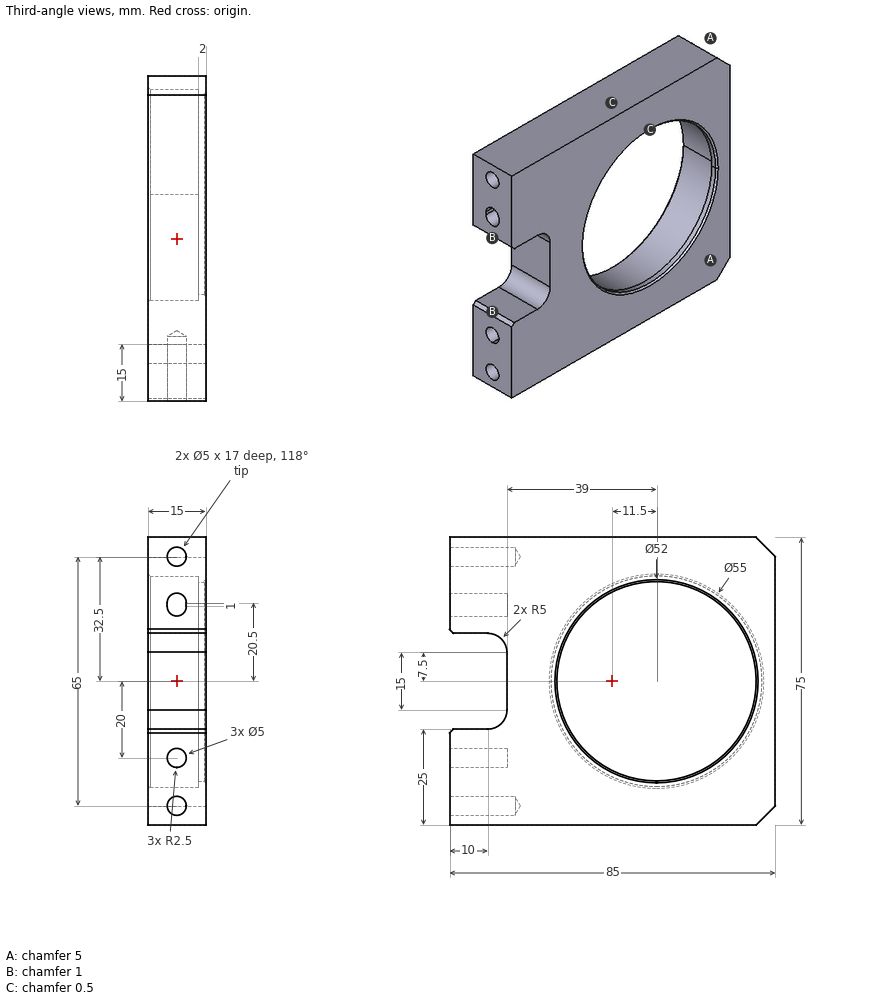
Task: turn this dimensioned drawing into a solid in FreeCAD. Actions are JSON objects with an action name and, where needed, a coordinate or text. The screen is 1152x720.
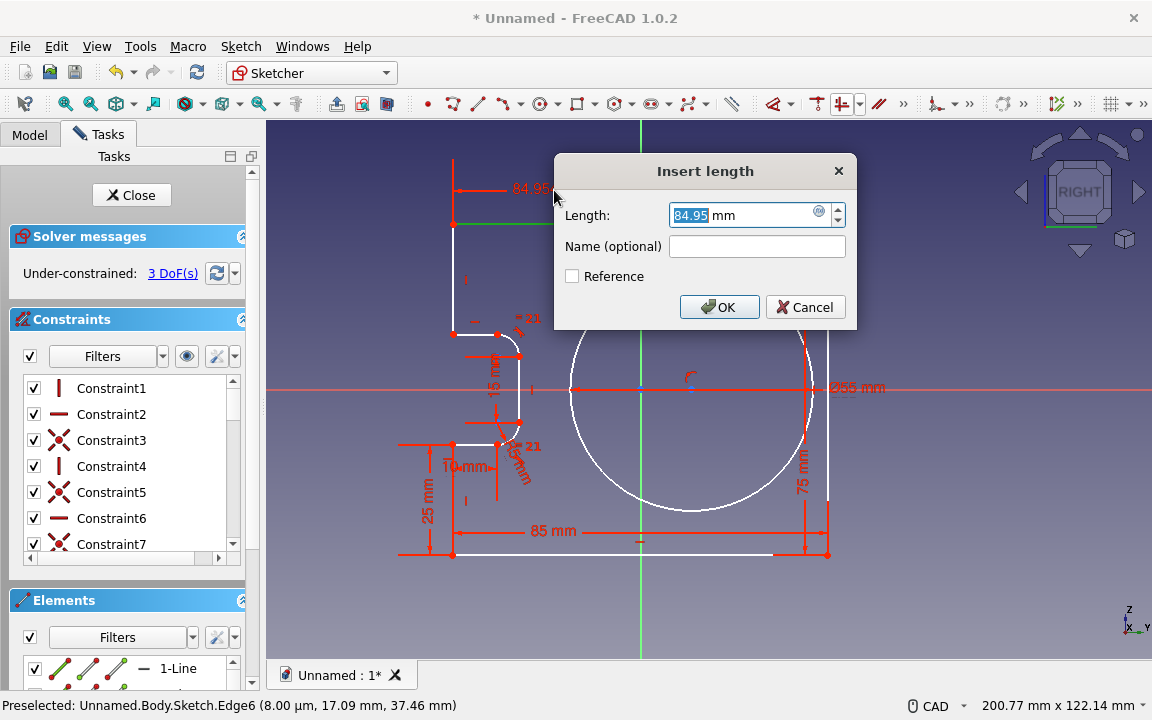
{"action": "type", "text": "85"}
{"action": "key", "text": "Return"}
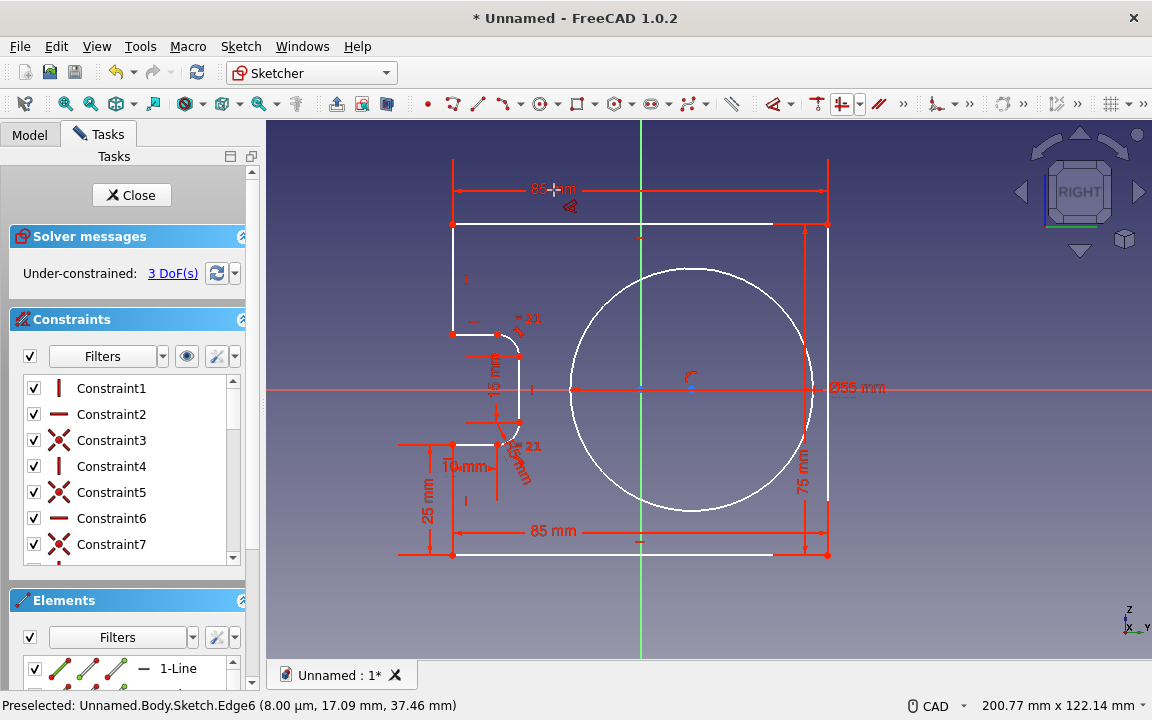
{"action": "left_click", "coordinate": [519, 357]}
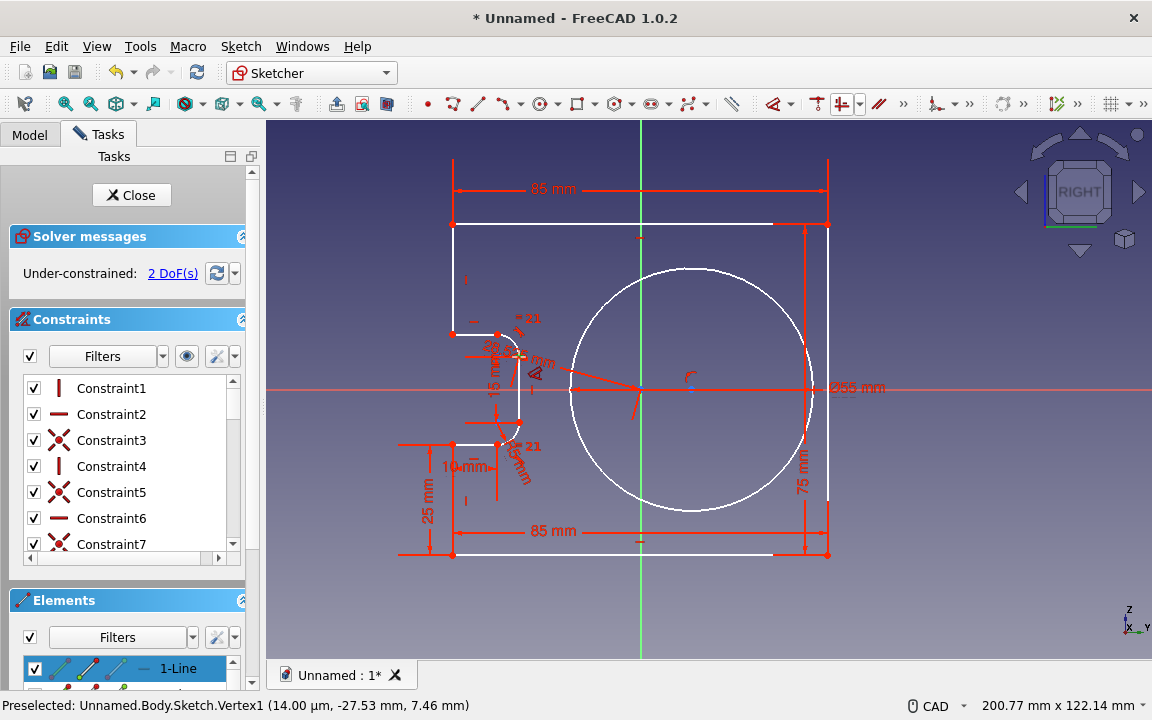
{"action": "left_click", "coordinate": [692, 390]}
{"action": "left_click", "coordinate": [566, 323]}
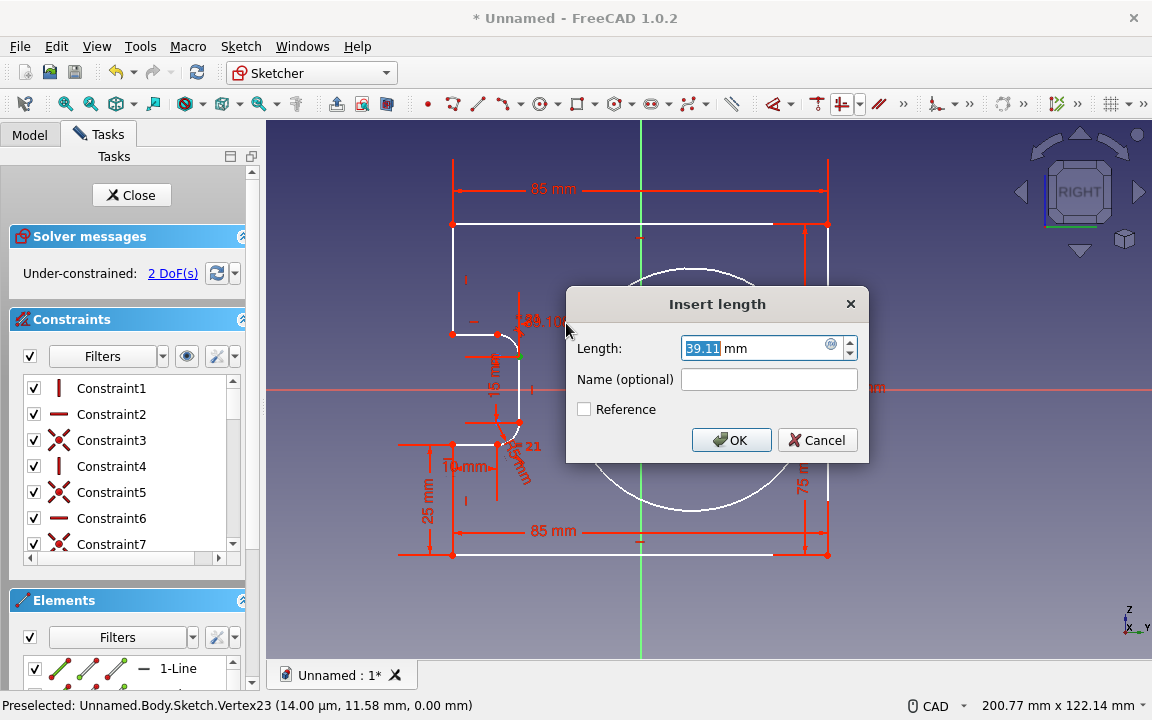
{"action": "type", "text": "39"}
{"action": "key", "text": "Return"}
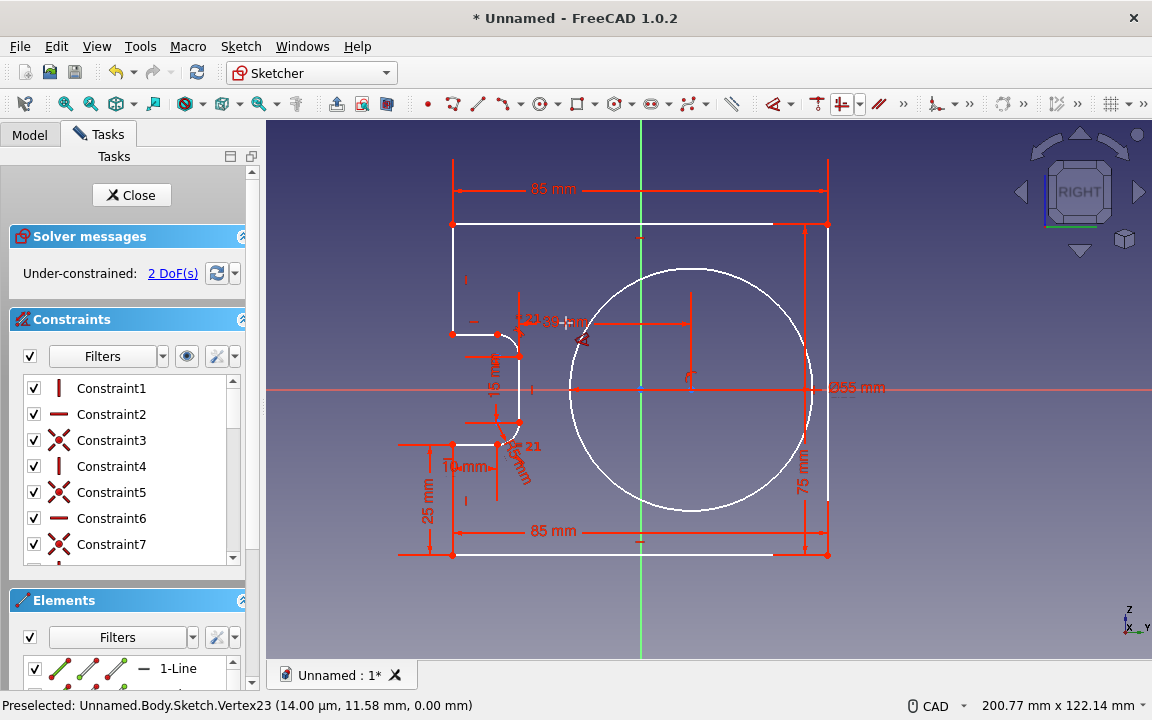
{"action": "left_click", "coordinate": [519, 357]}
{"action": "left_click", "coordinate": [675, 373]}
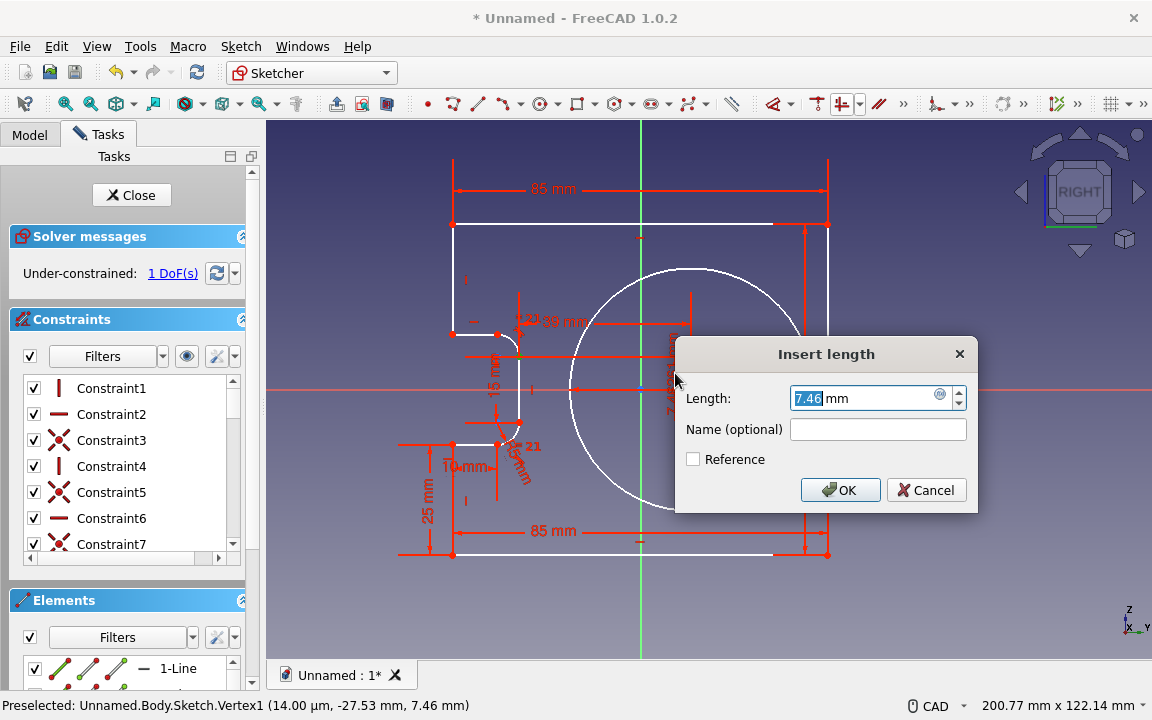
{"action": "type", "text": "7.5"}
{"action": "key", "text": "Return"}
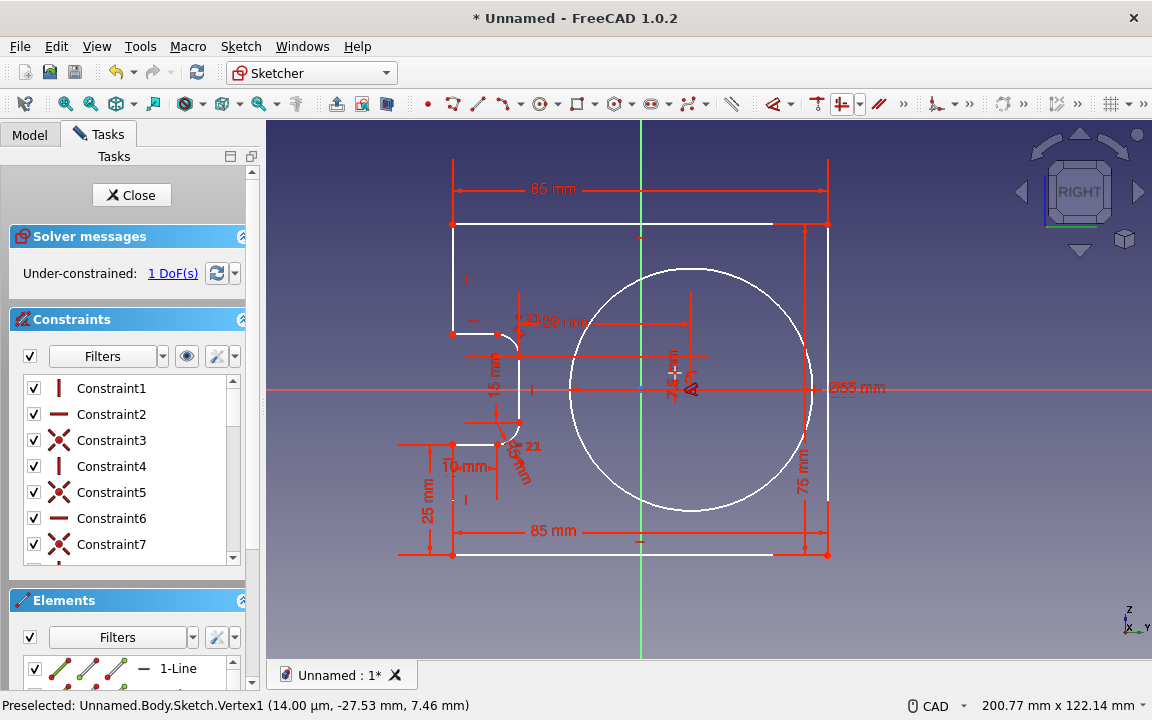
{"action": "left_click", "coordinate": [691, 390]}
{"action": "left_click", "coordinate": [666, 424]}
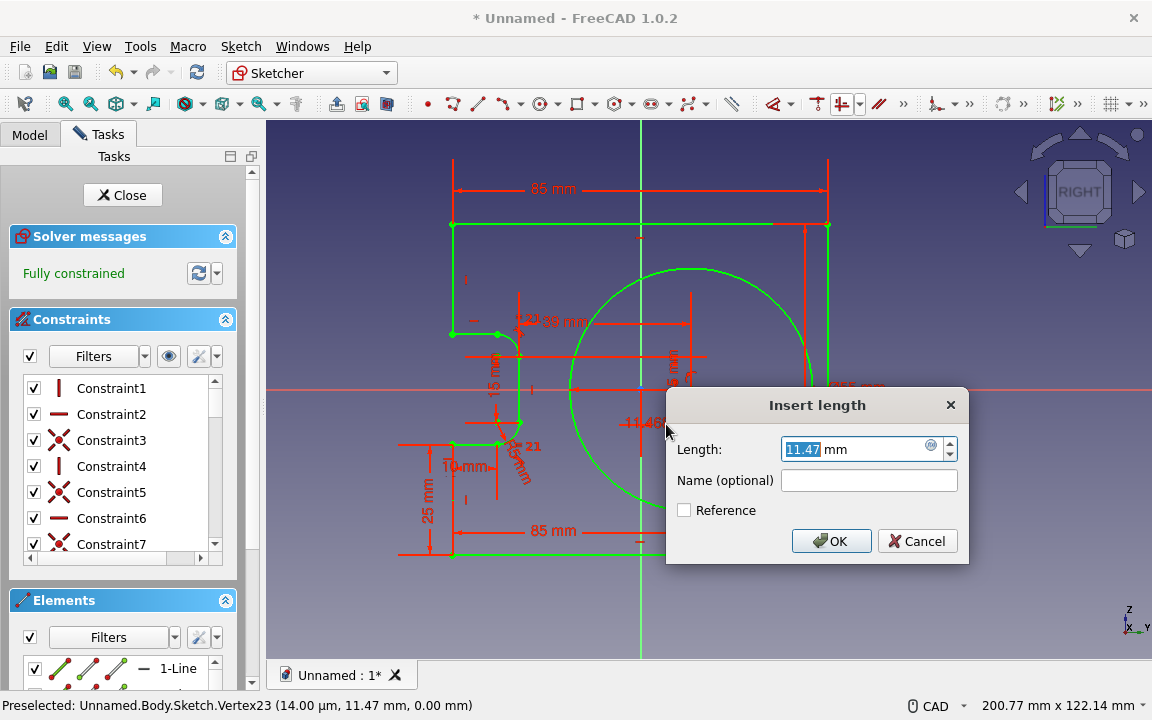
{"action": "type", "text": "11.5"}
{"action": "key", "text": "Return"}
{"action": "key", "text": "Escape"}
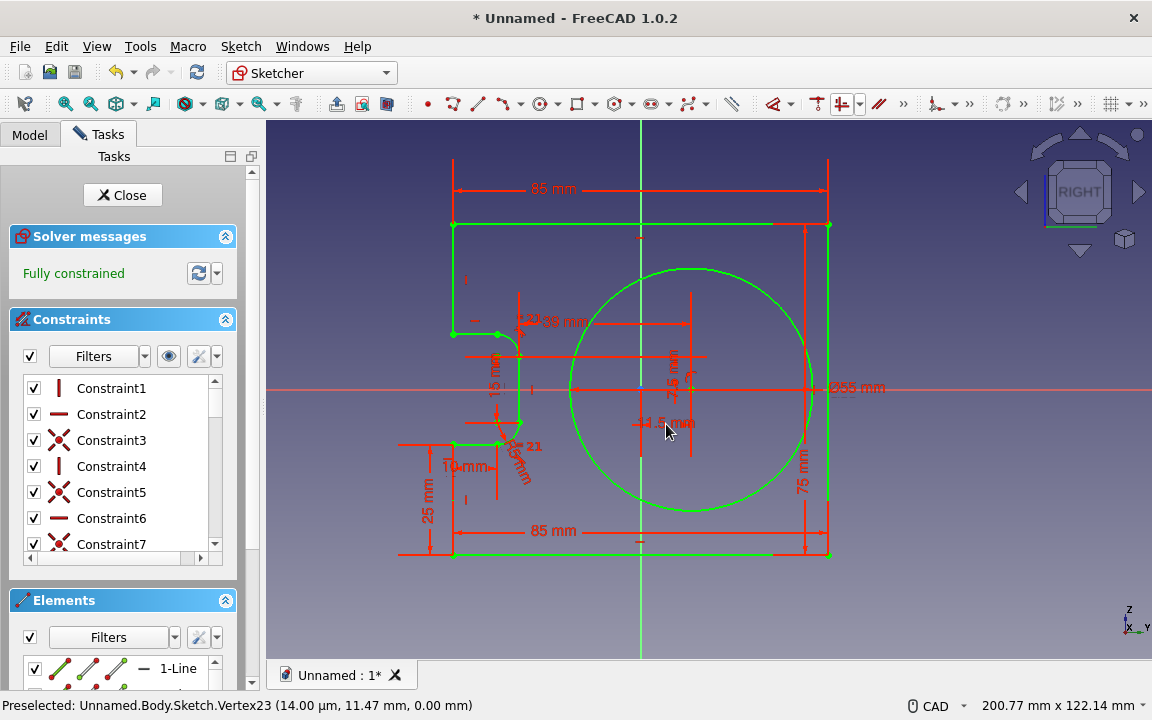
{"action": "left_click", "coordinate": [123, 195]}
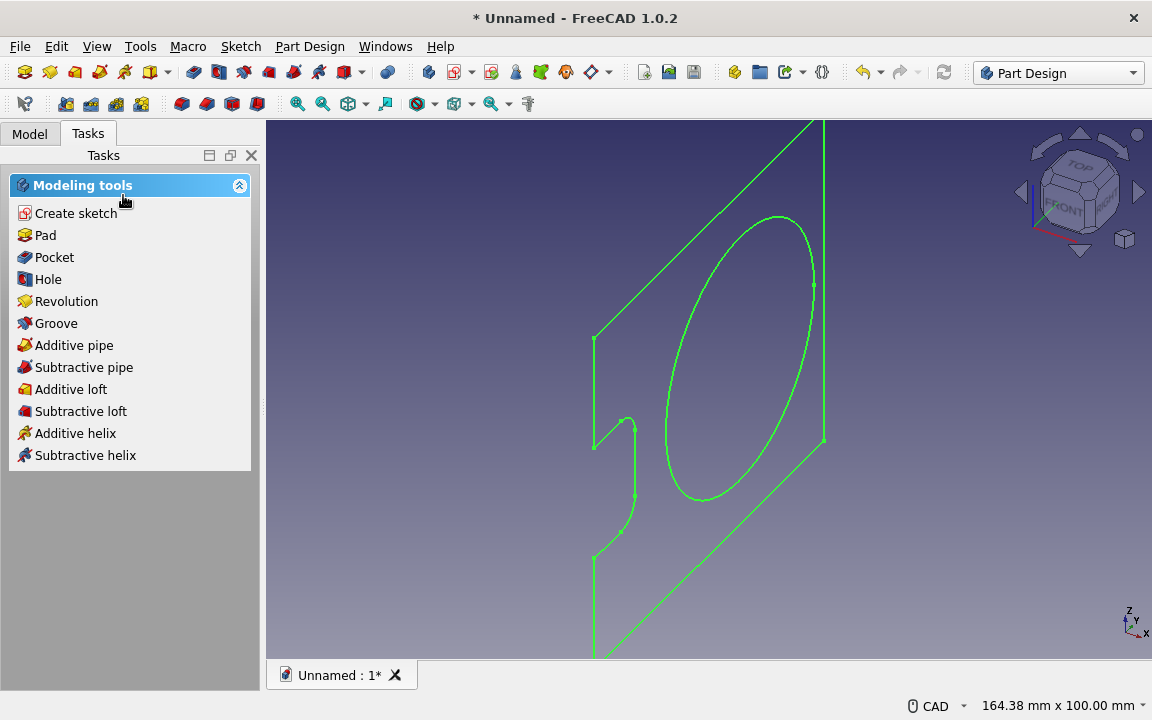
{"action": "left_click", "coordinate": [25, 72]}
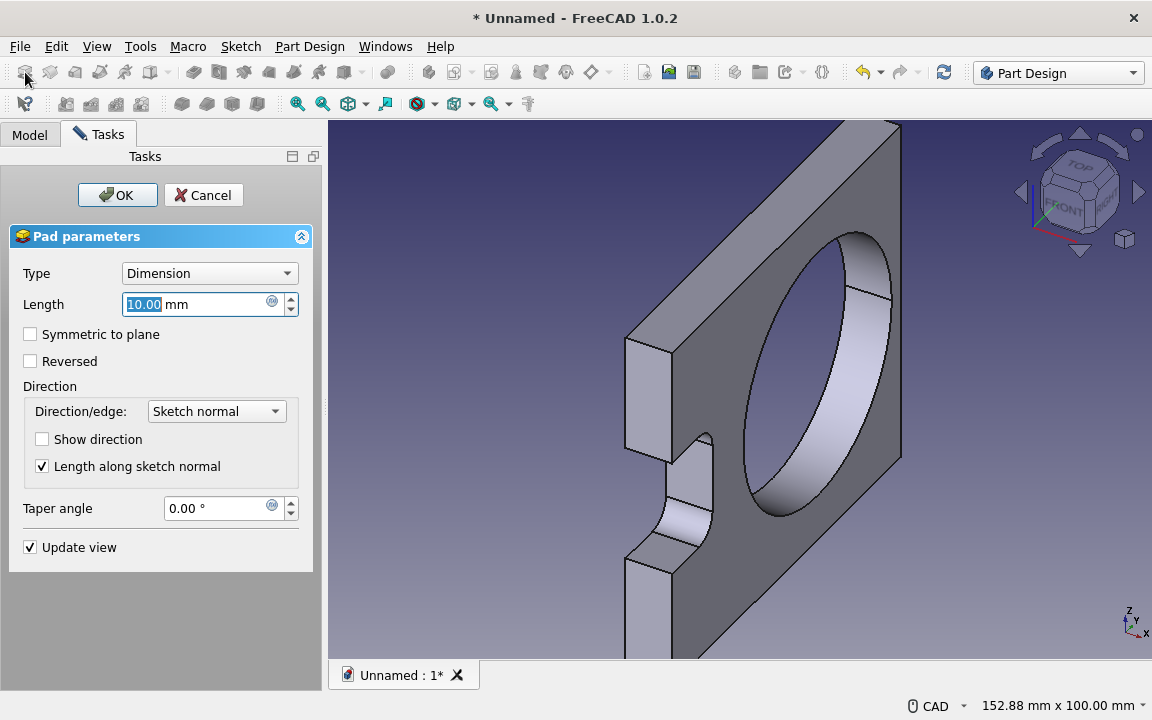
{"action": "type", "text": "15"}
{"action": "key", "text": "Tab"}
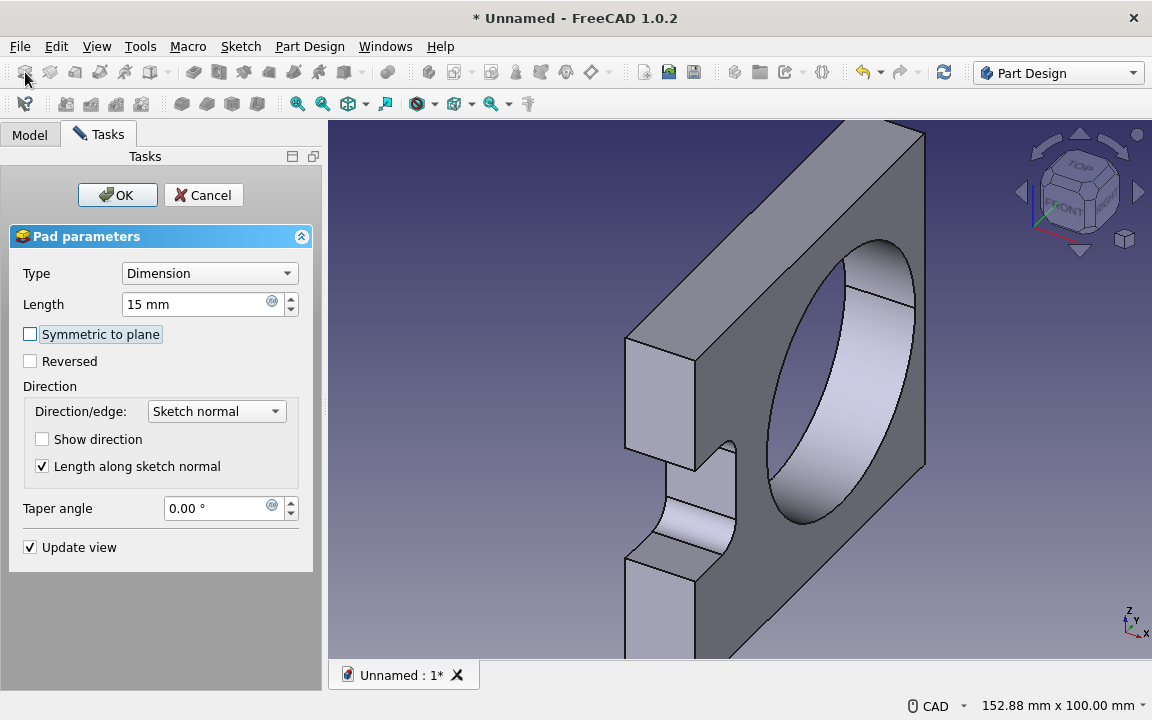
{"action": "left_click", "coordinate": [31, 334]}